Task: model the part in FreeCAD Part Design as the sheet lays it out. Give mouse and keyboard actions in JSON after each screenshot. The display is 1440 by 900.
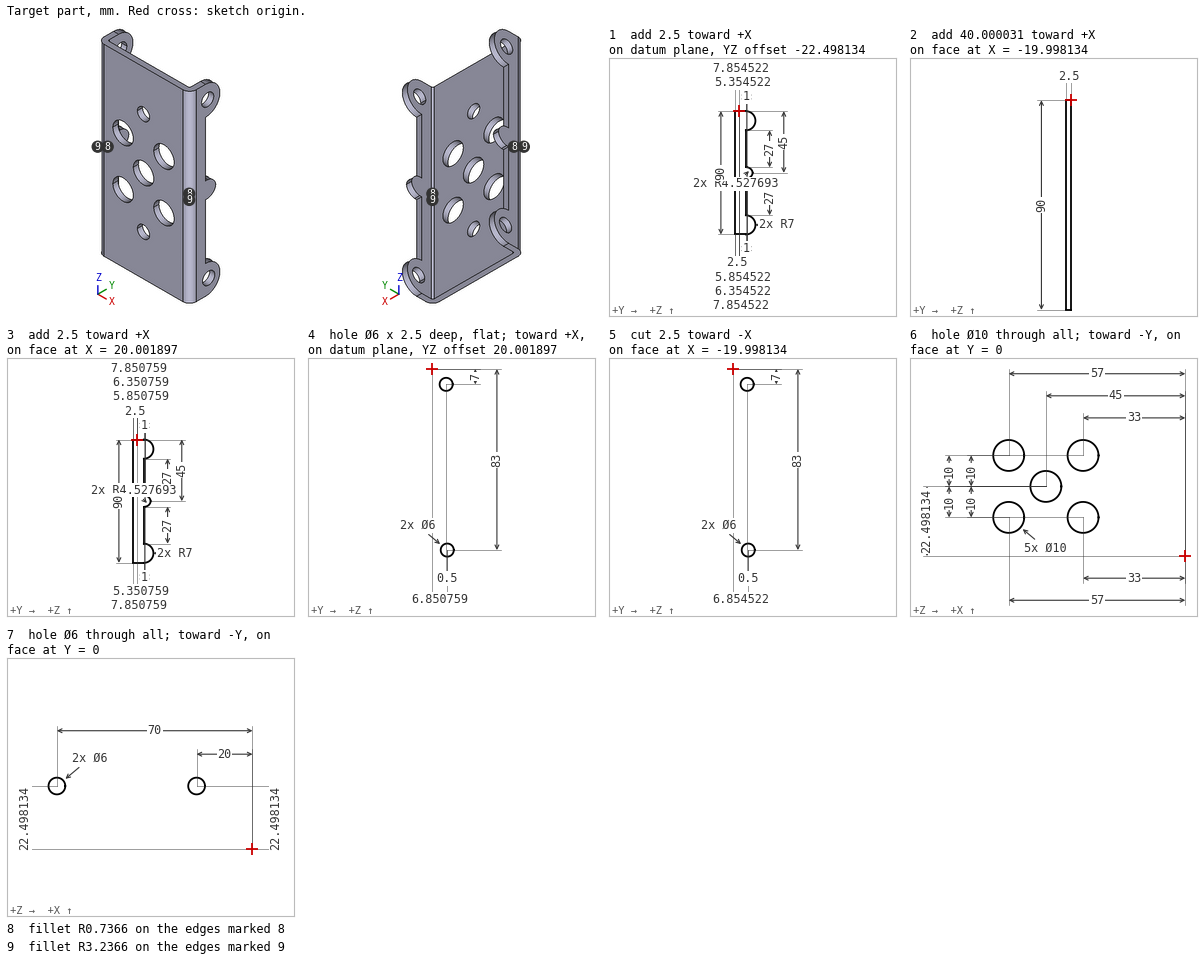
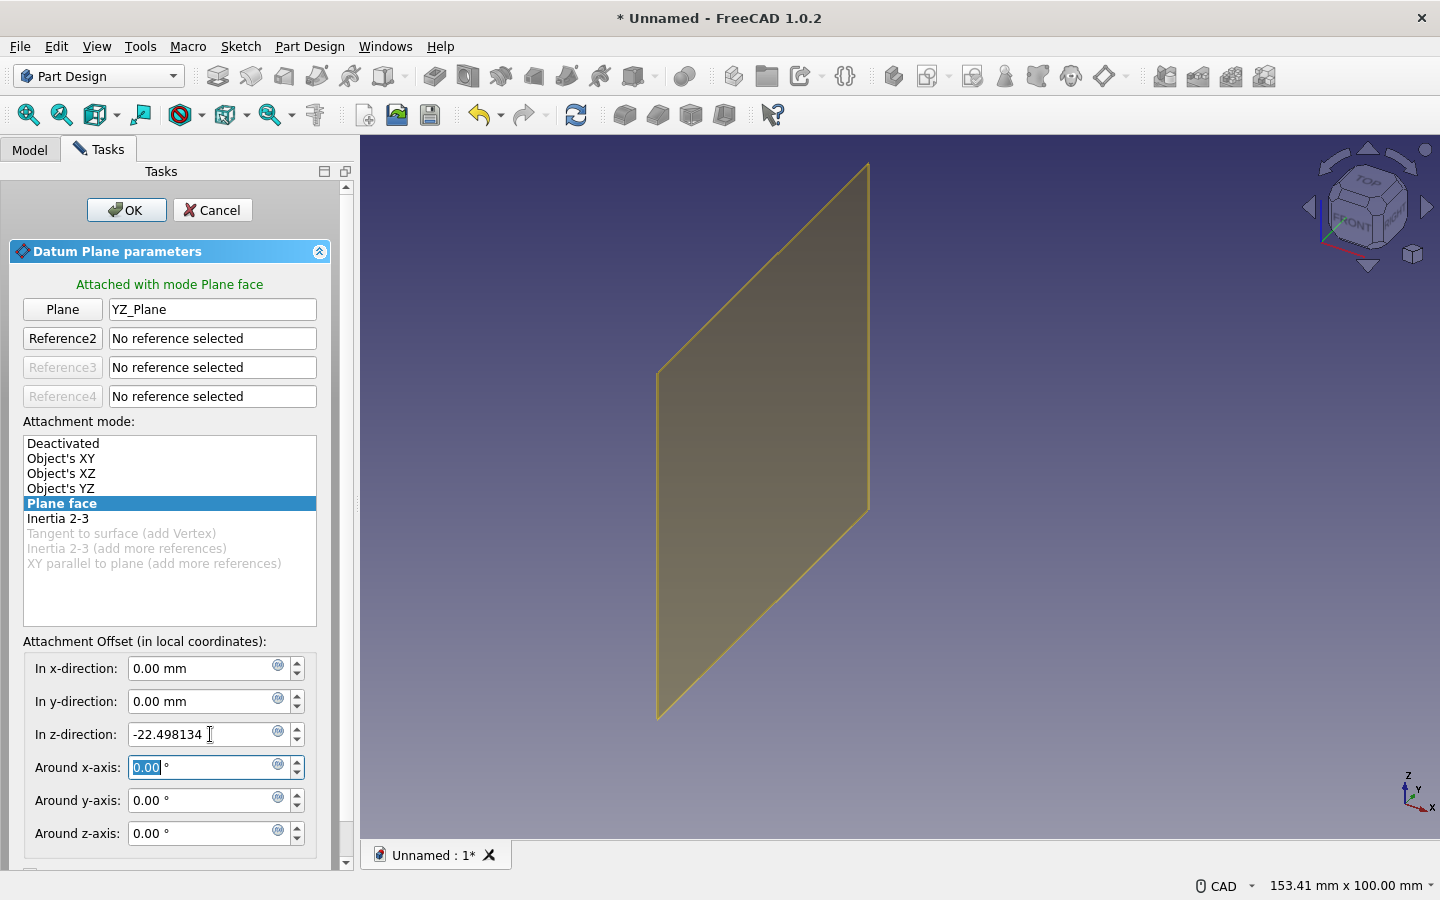
{"action": "left_click", "coordinate": [127, 210]}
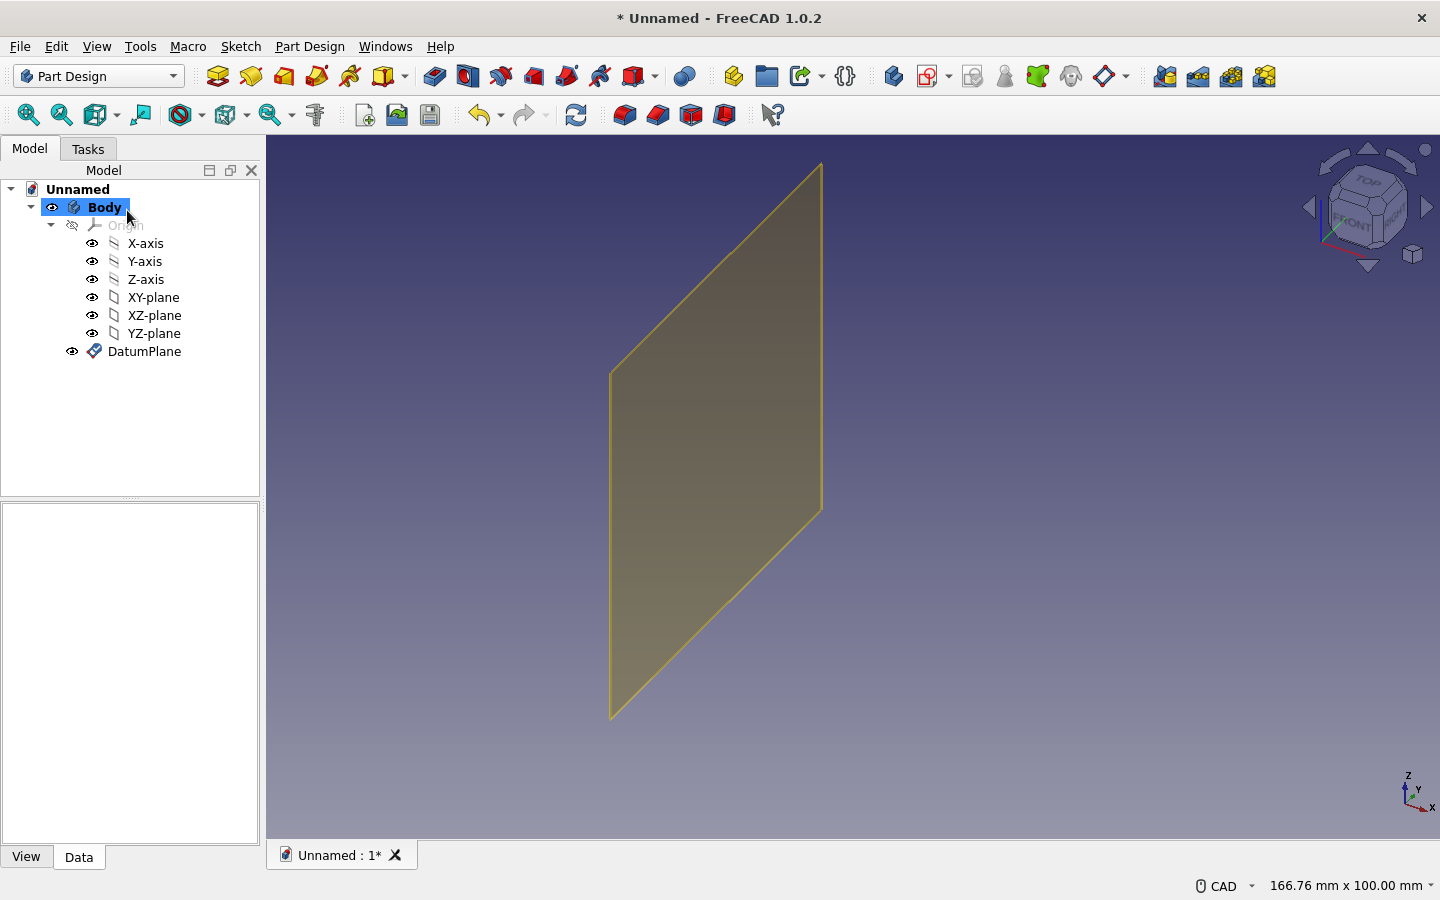
{"action": "left_click", "coordinate": [117, 351]}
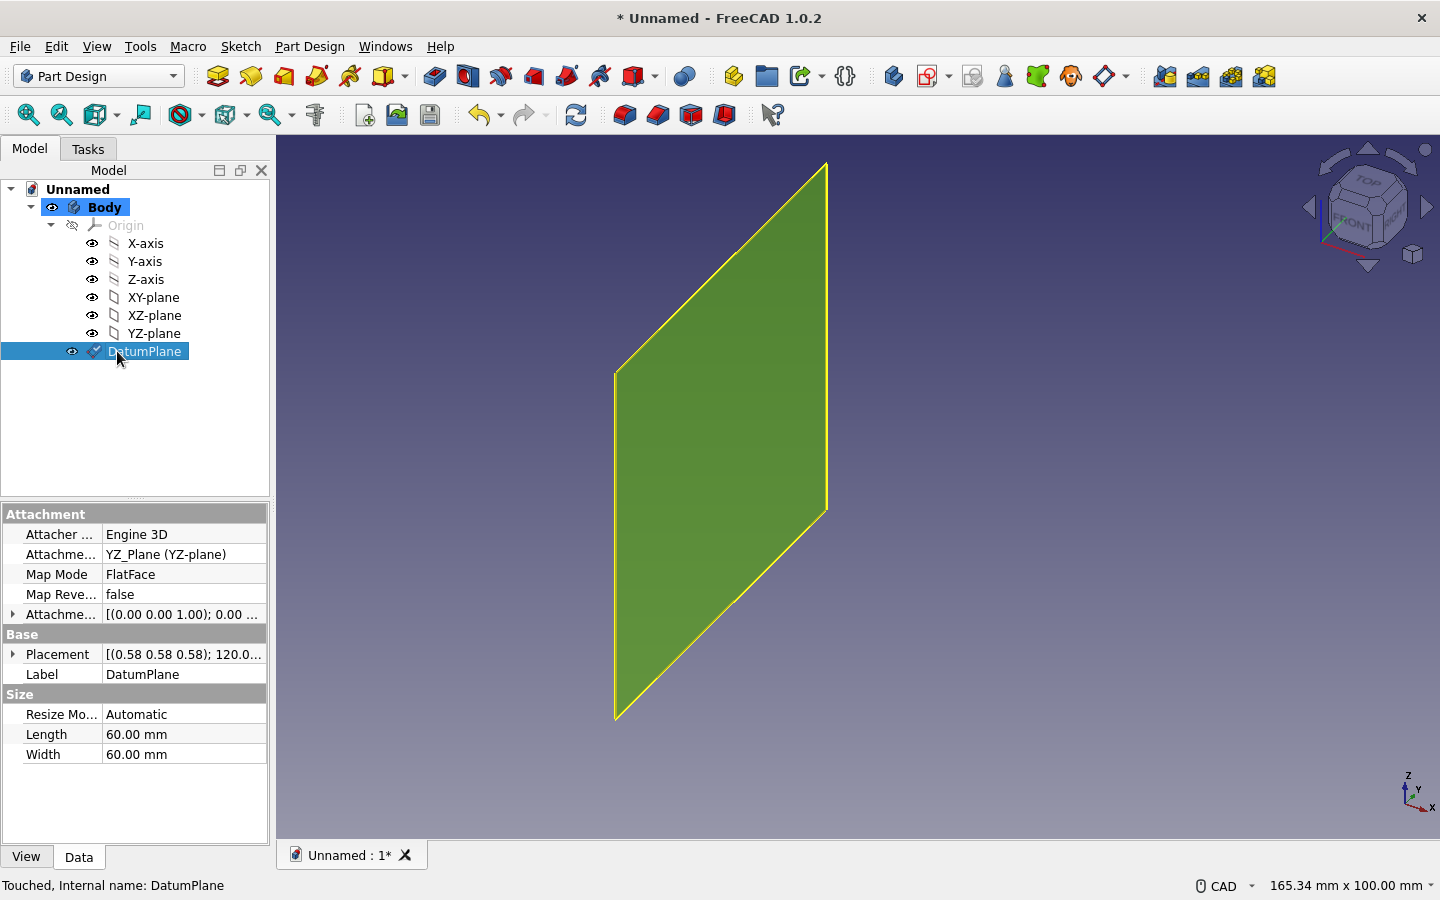
{"action": "left_click", "coordinate": [926, 76]}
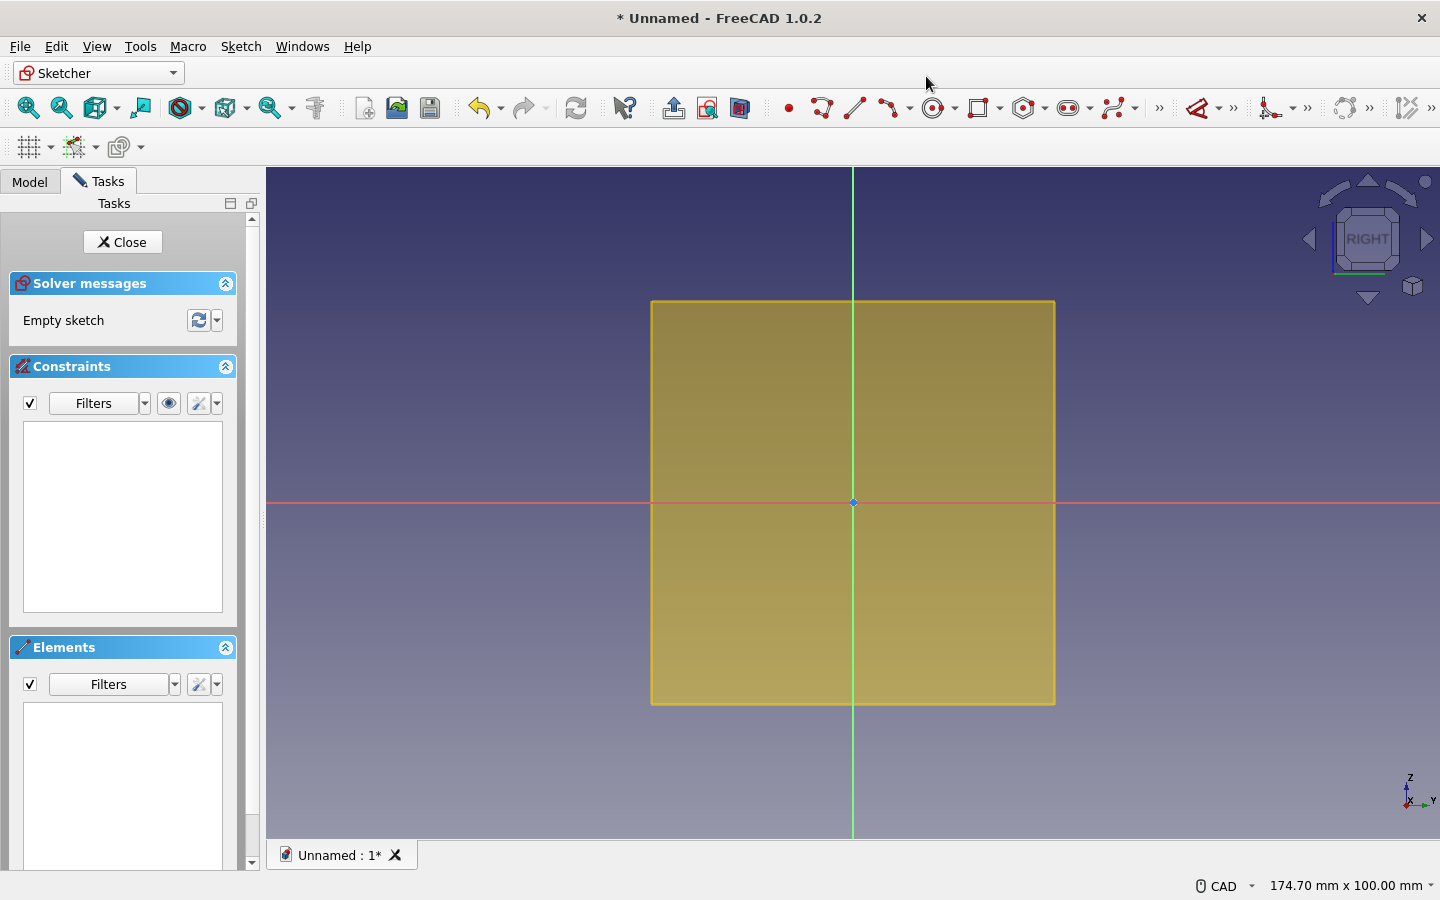
{"action": "scroll", "coordinate": [661, 195], "scroll_direction": "down", "scroll_amount": 3}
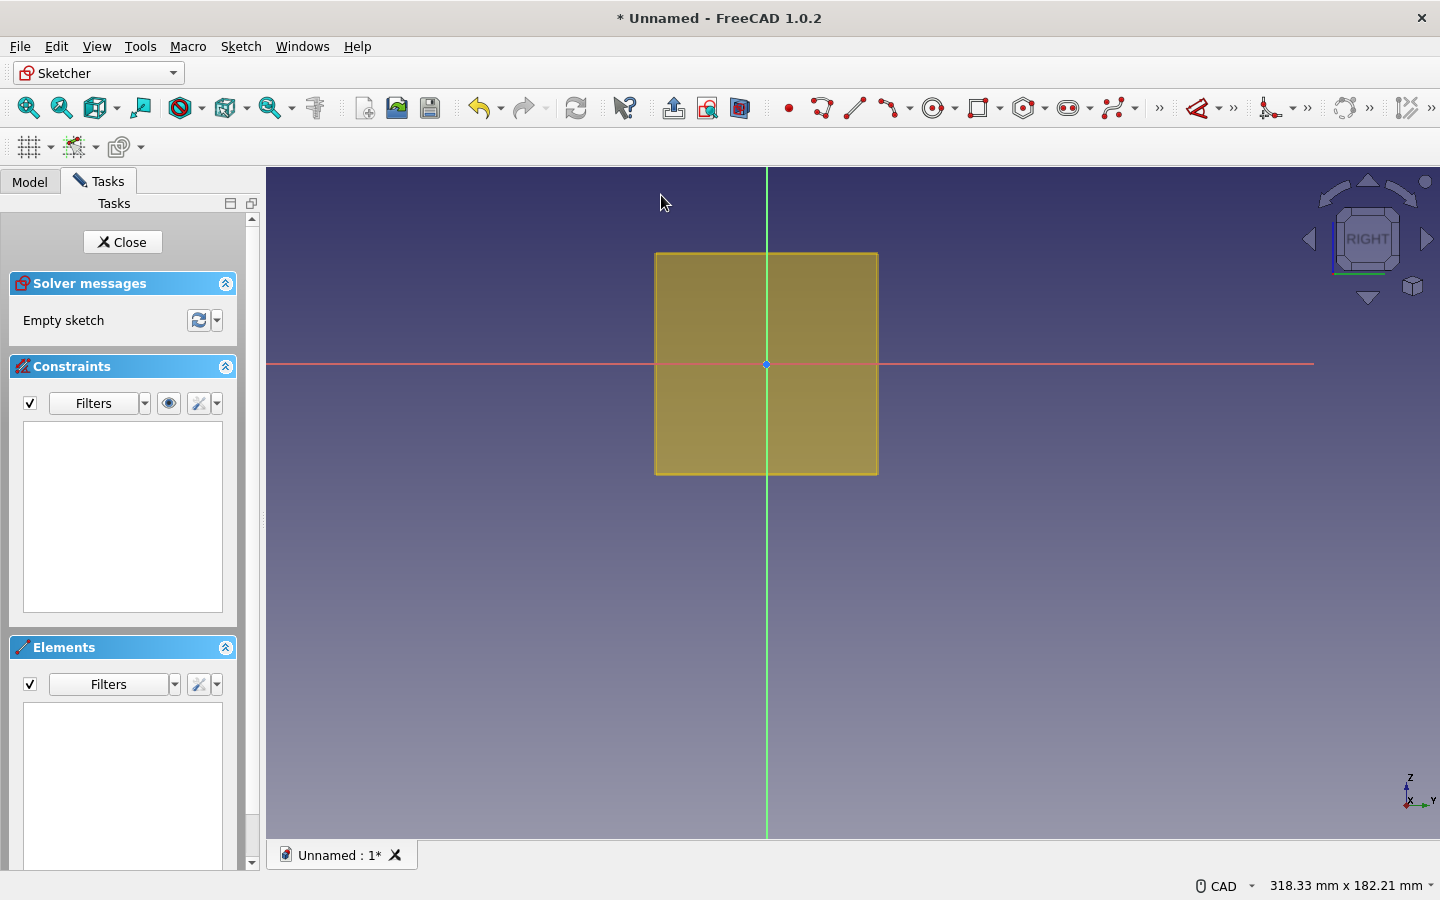
{"action": "left_click", "coordinate": [822, 108]}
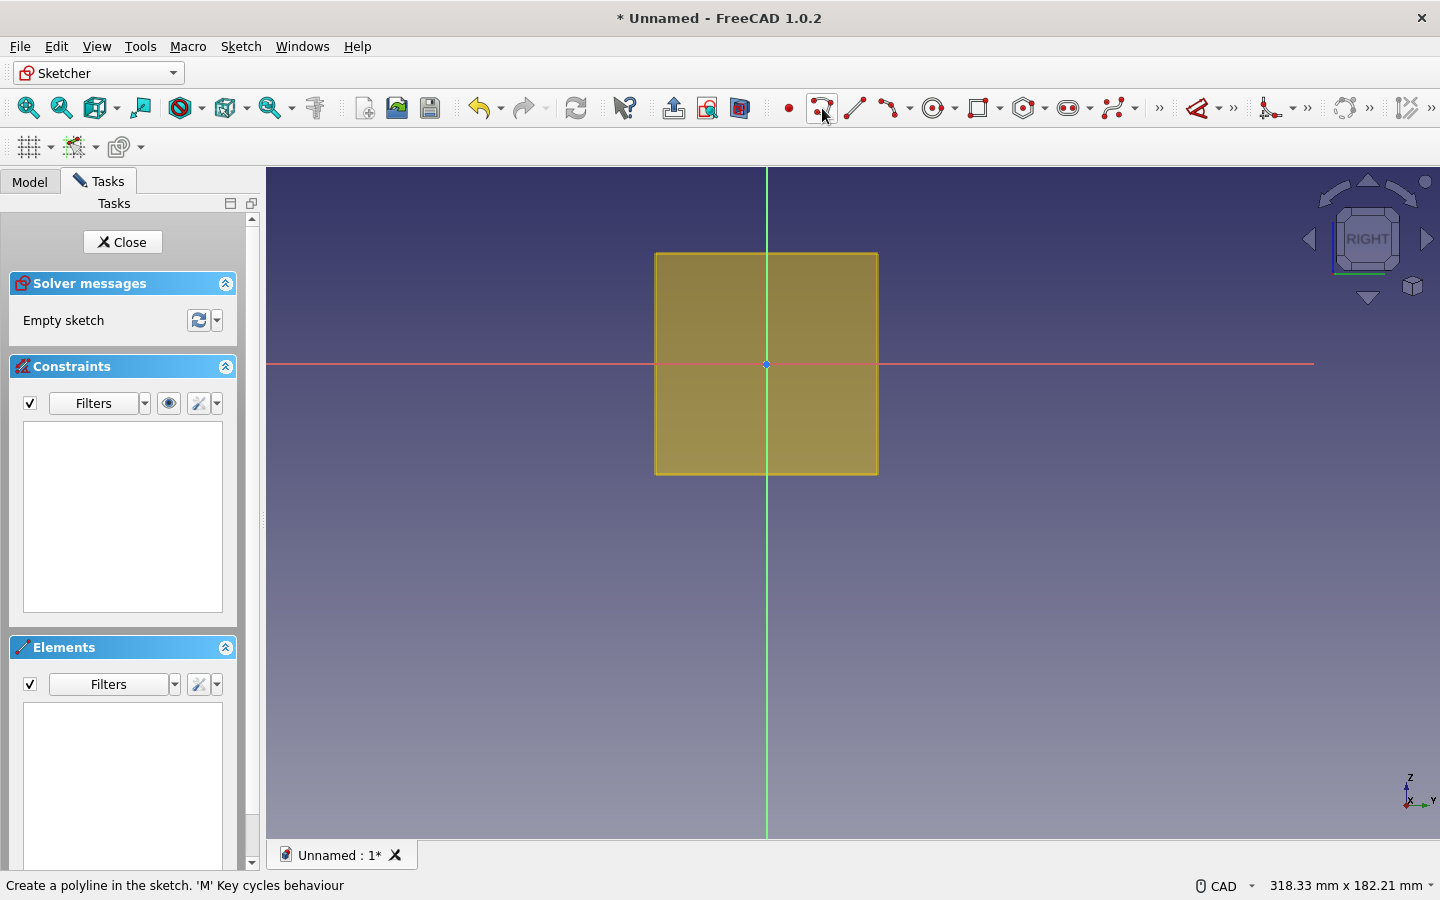
{"action": "left_click", "coordinate": [786, 696]}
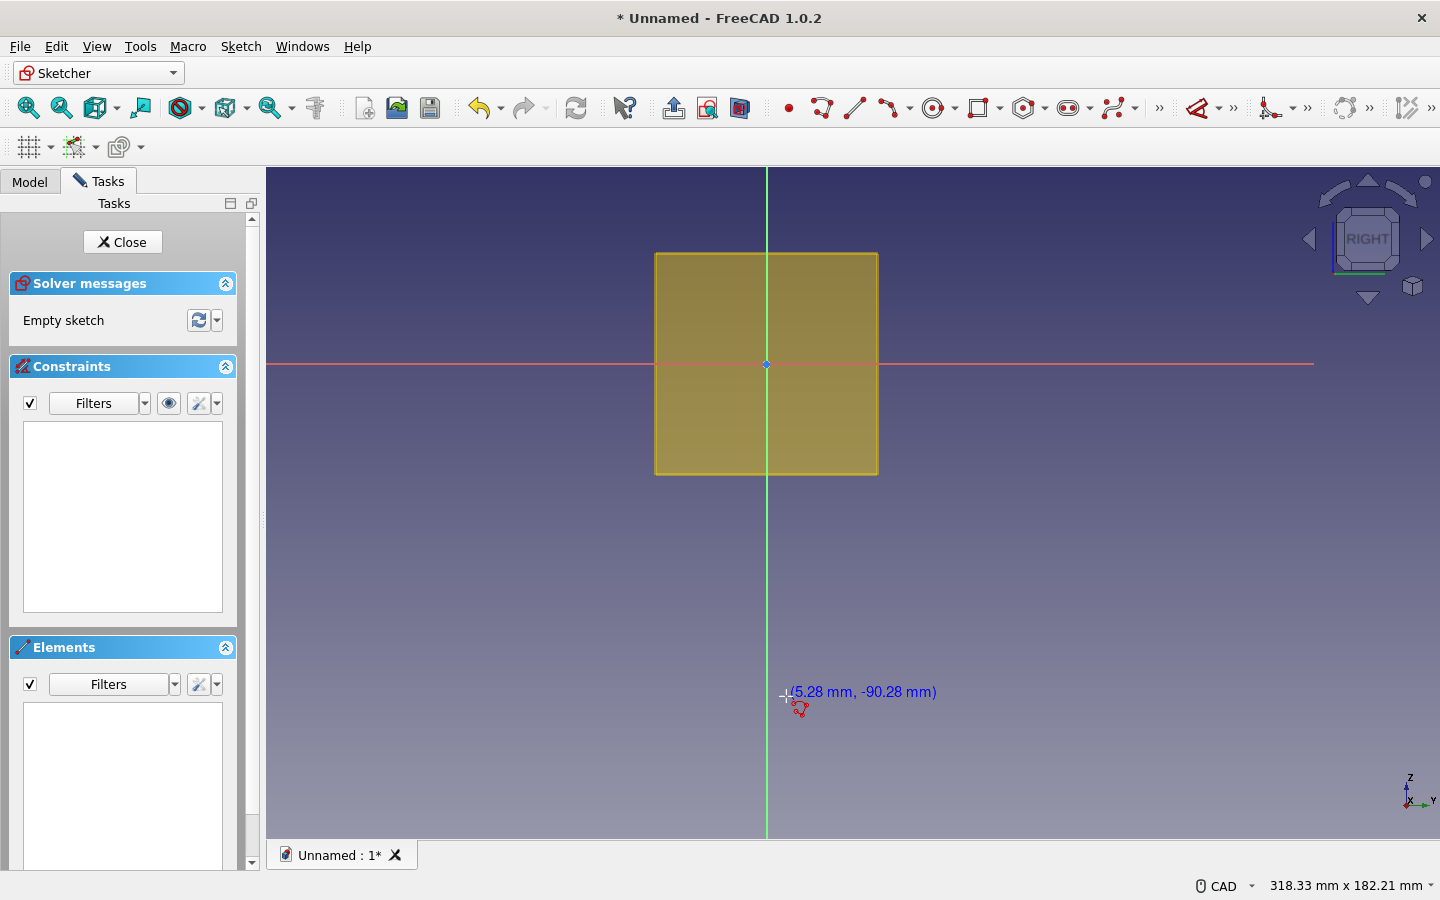
{"action": "scroll", "coordinate": [757, 696], "scroll_direction": "up", "scroll_amount": 3}